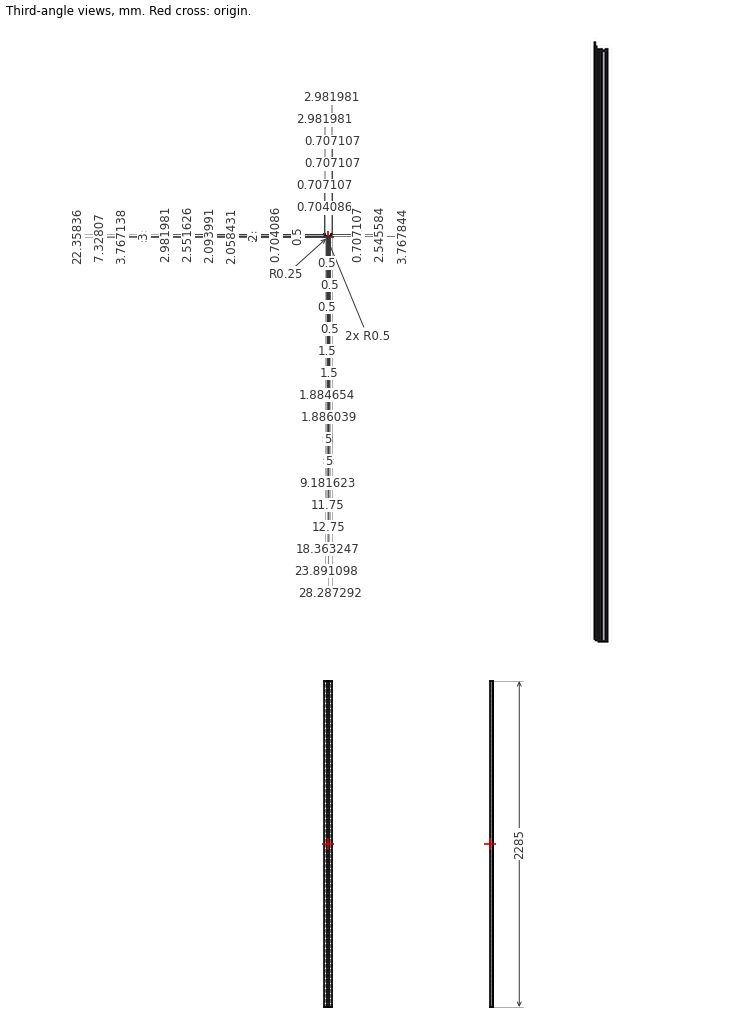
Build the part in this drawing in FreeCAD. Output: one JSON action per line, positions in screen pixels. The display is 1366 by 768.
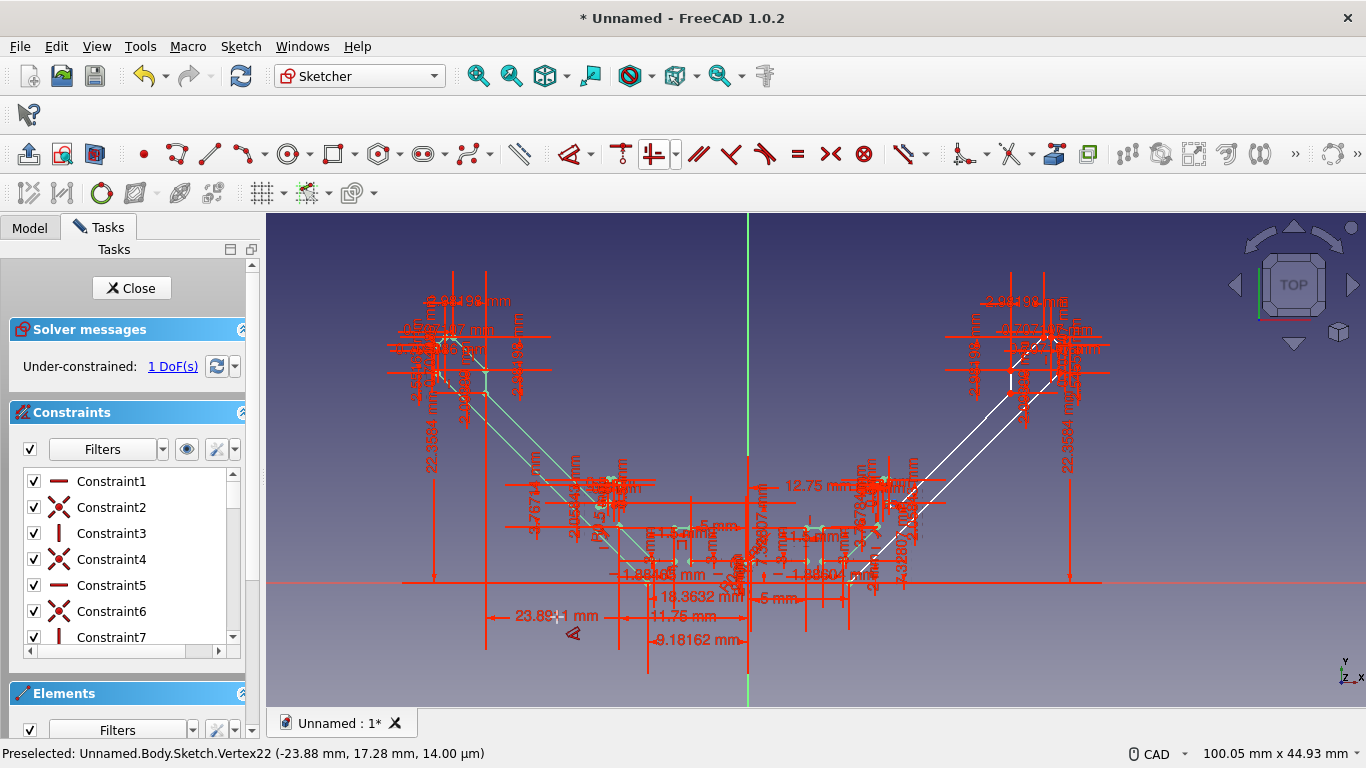
{"action": "left_click", "coordinate": [1059, 373]}
{"action": "left_click", "coordinate": [904, 617]}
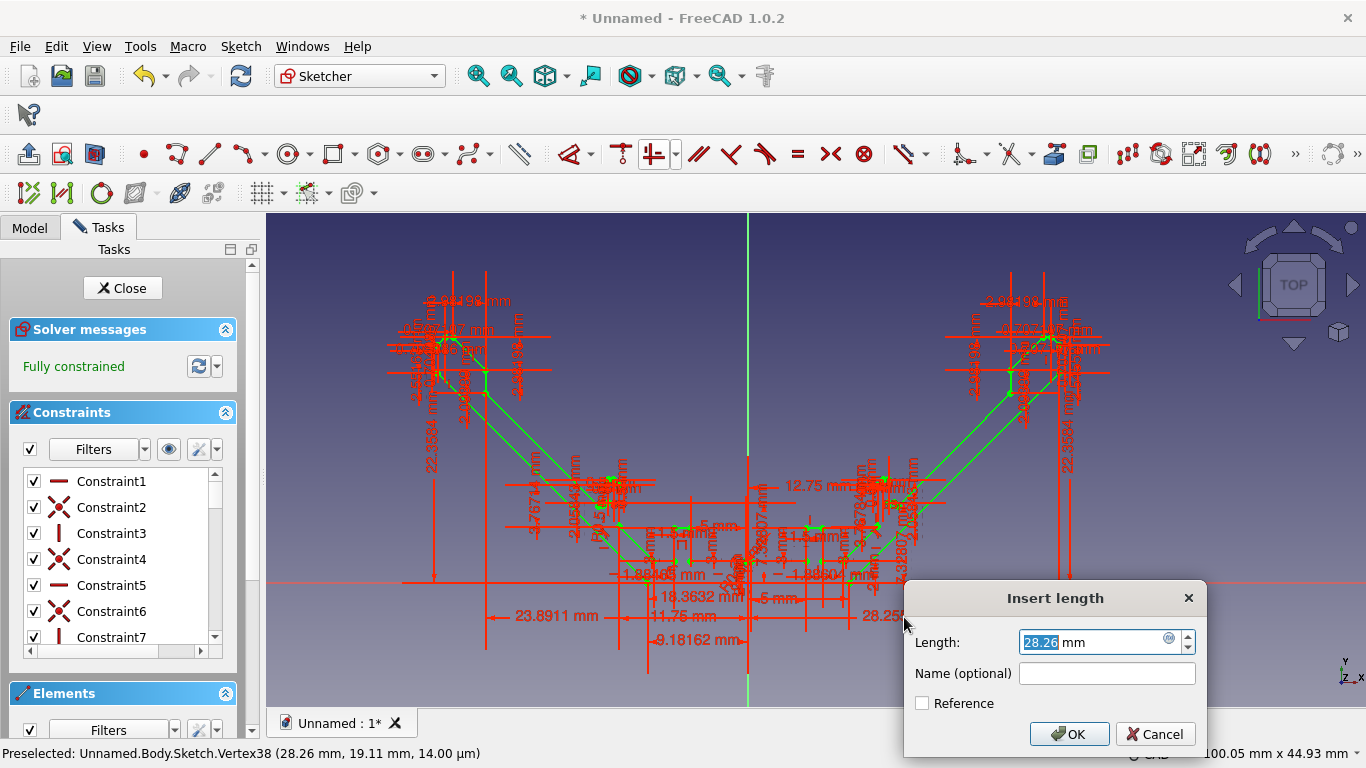
{"action": "type", "text": "28.287292"}
{"action": "key", "text": "Return"}
{"action": "key", "text": "Escape"}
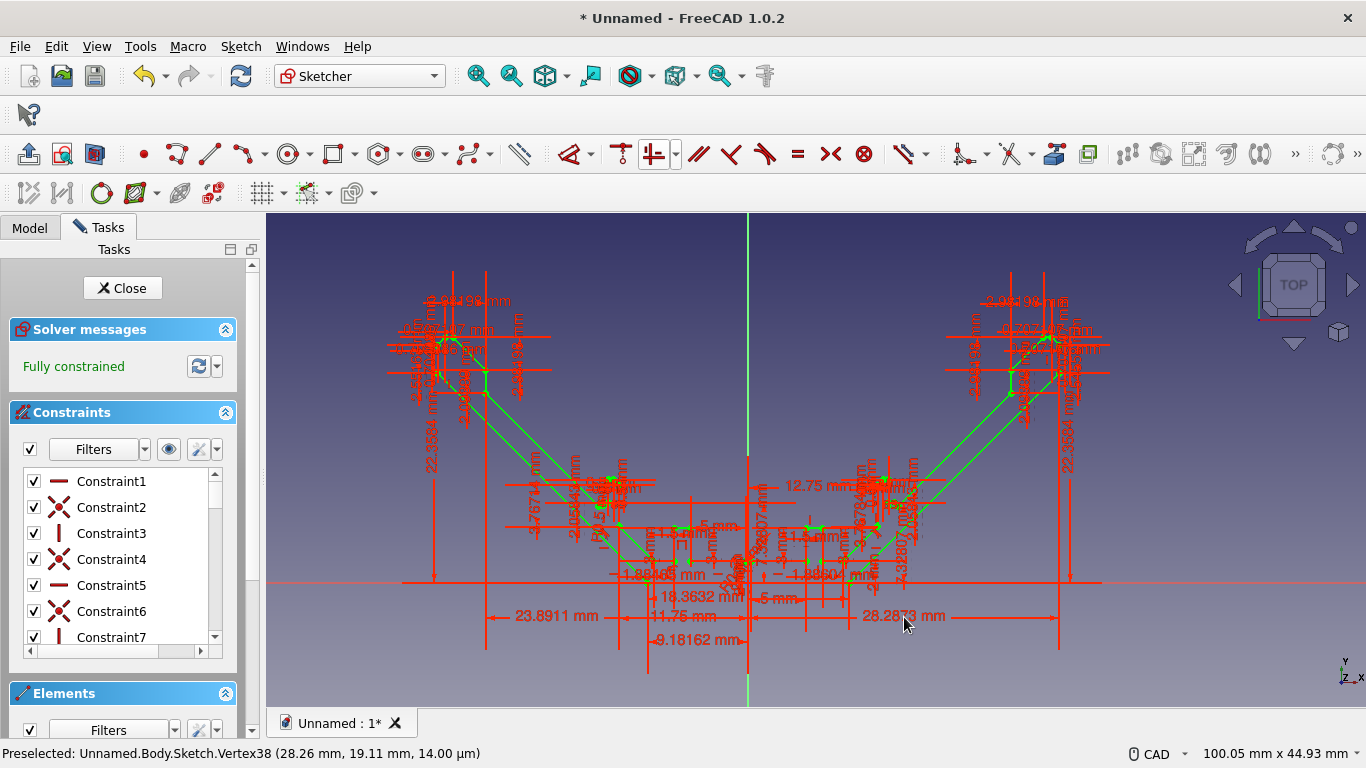
{"action": "left_click", "coordinate": [123, 288]}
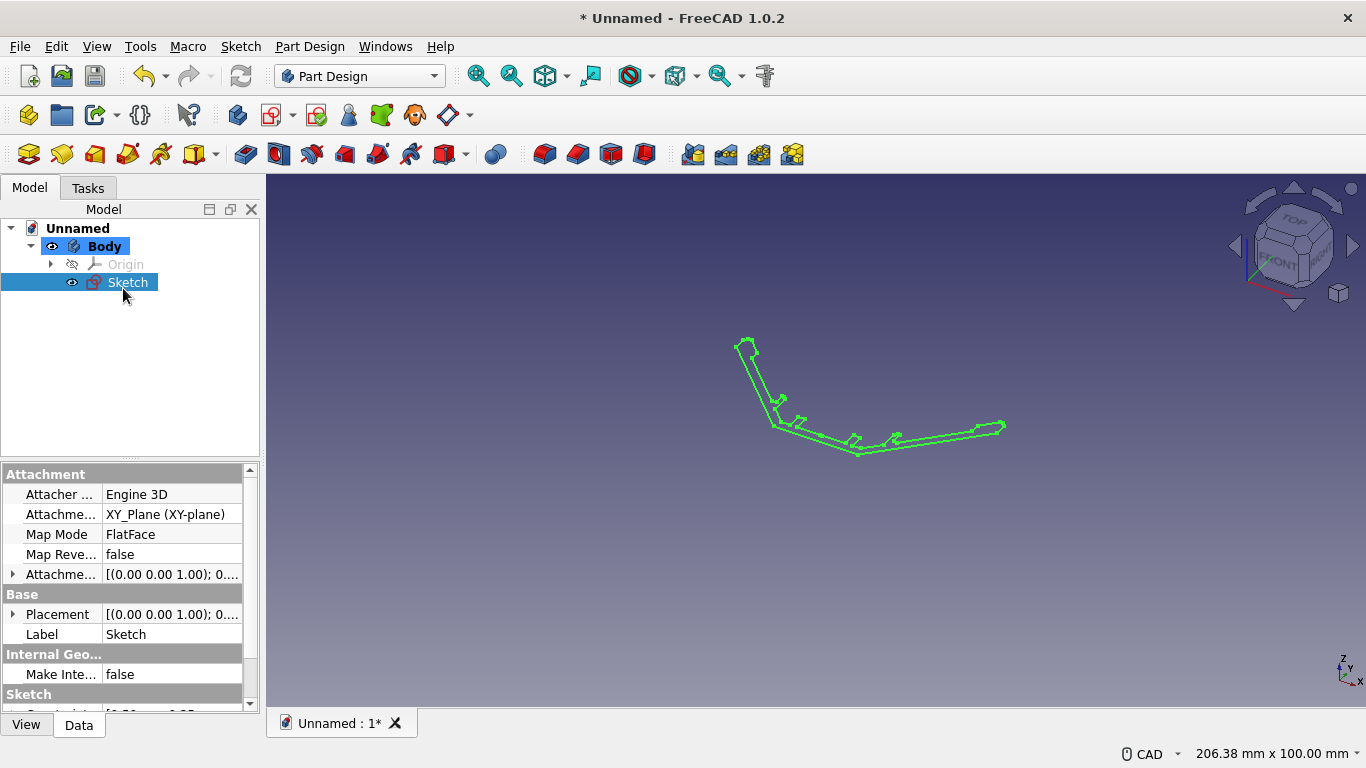
{"action": "left_click", "coordinate": [29, 154]}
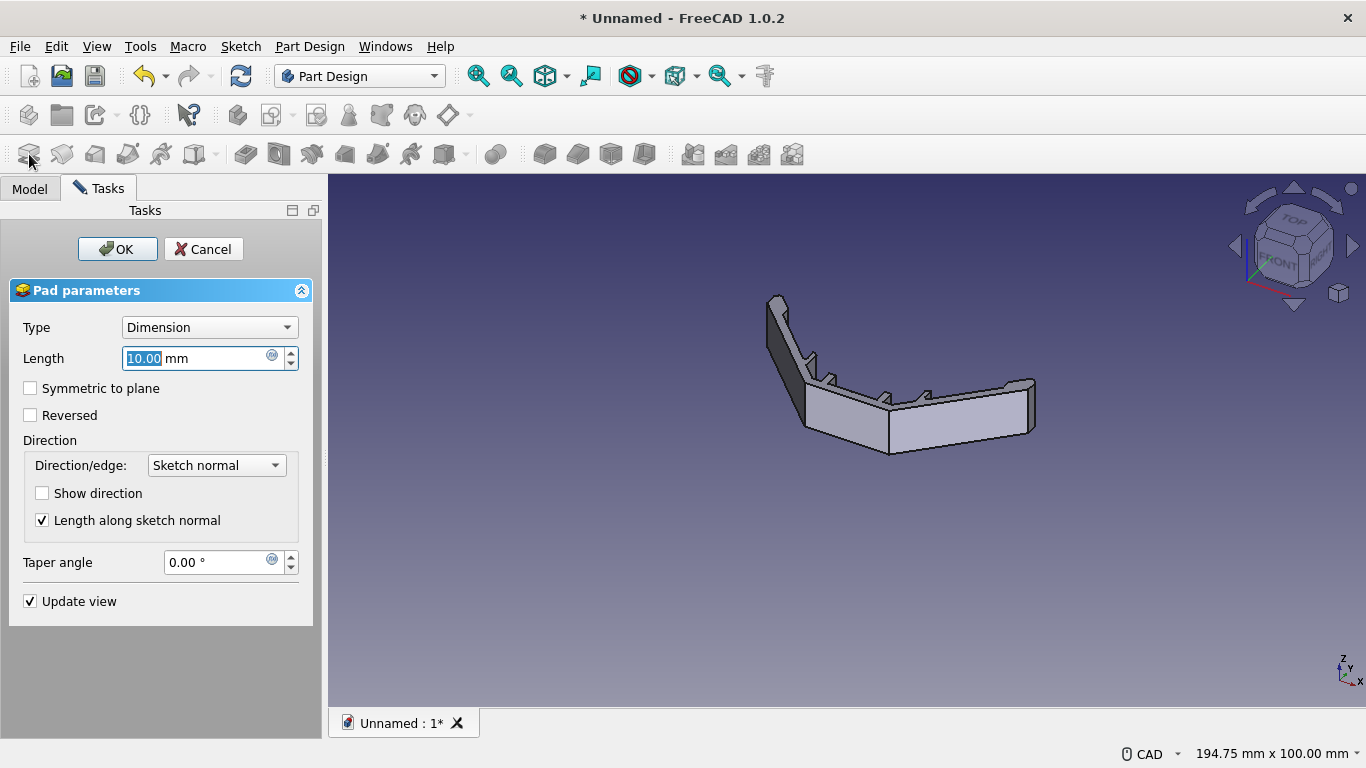
{"action": "type", "text": "2285"}
{"action": "key", "text": "Tab"}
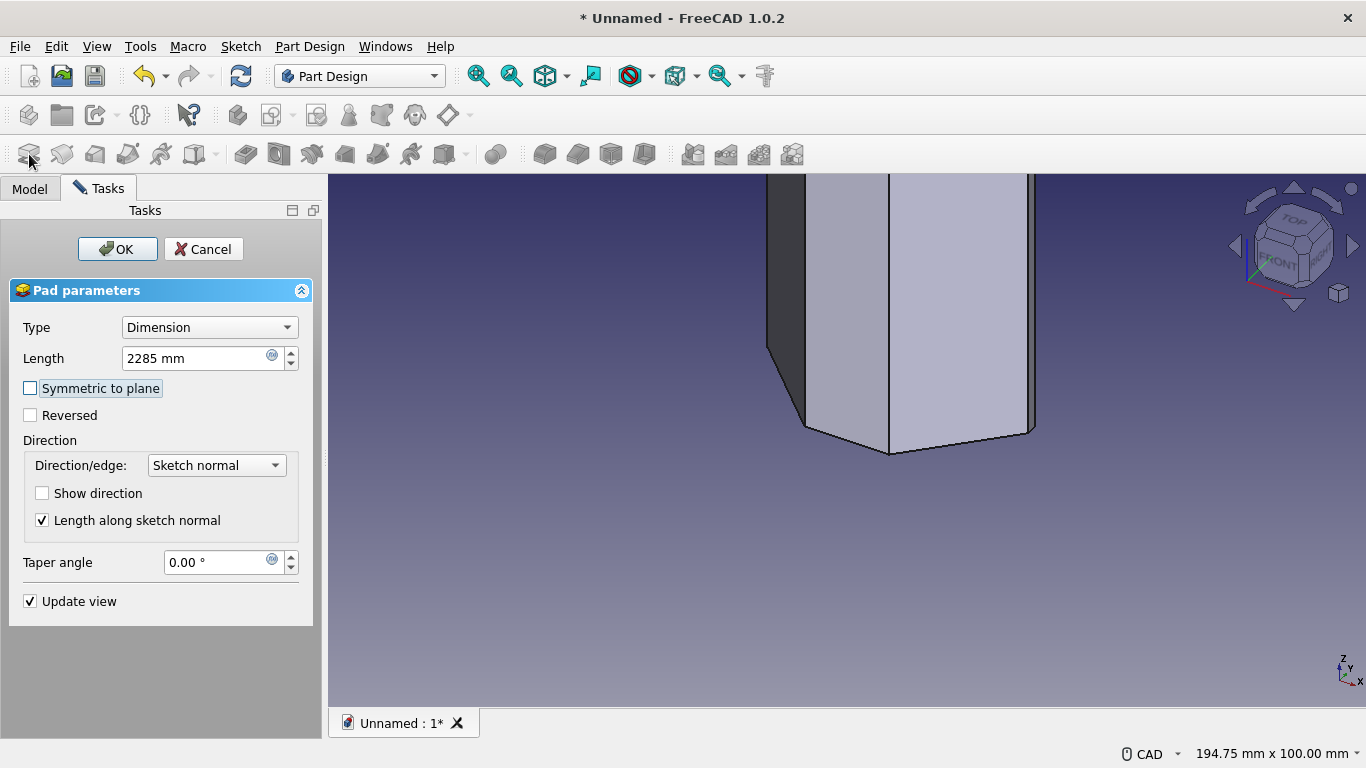
{"action": "left_click", "coordinate": [31, 388]}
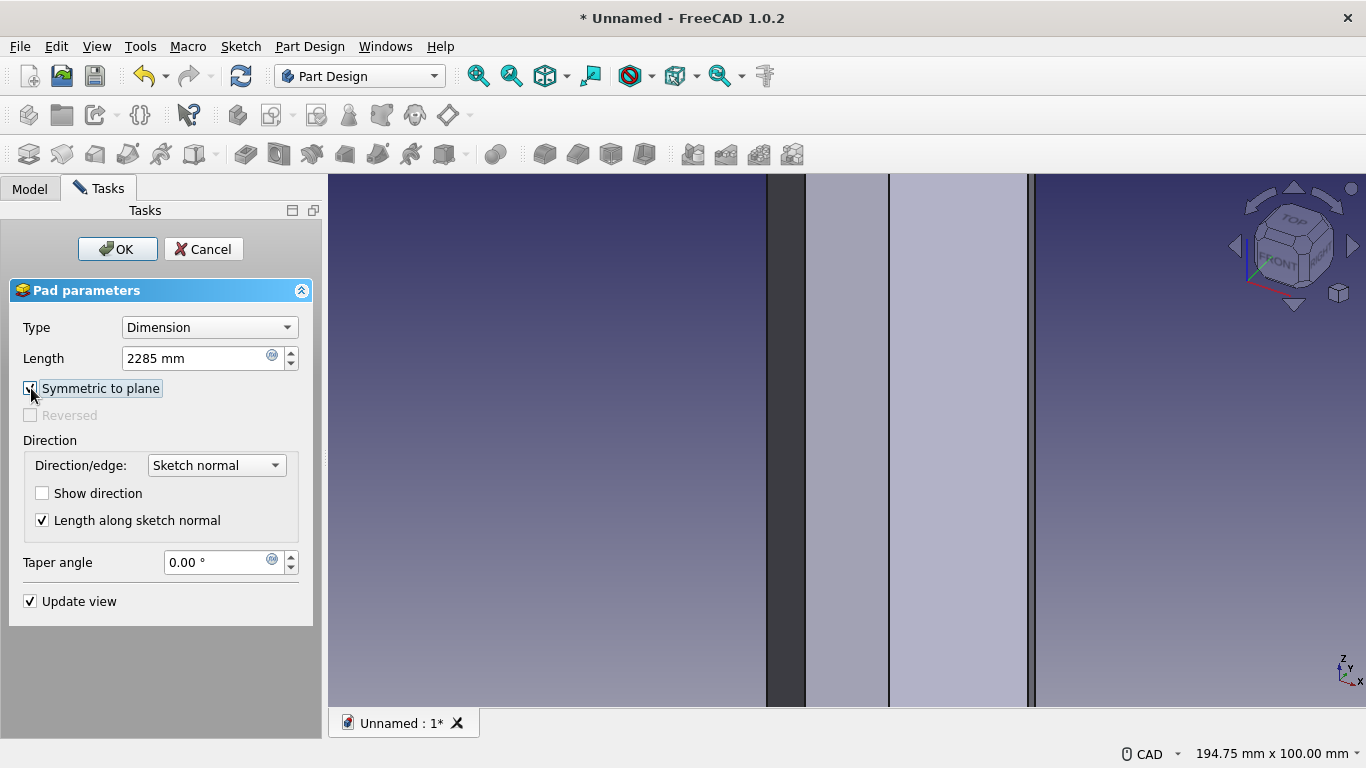
{"action": "left_click", "coordinate": [118, 249]}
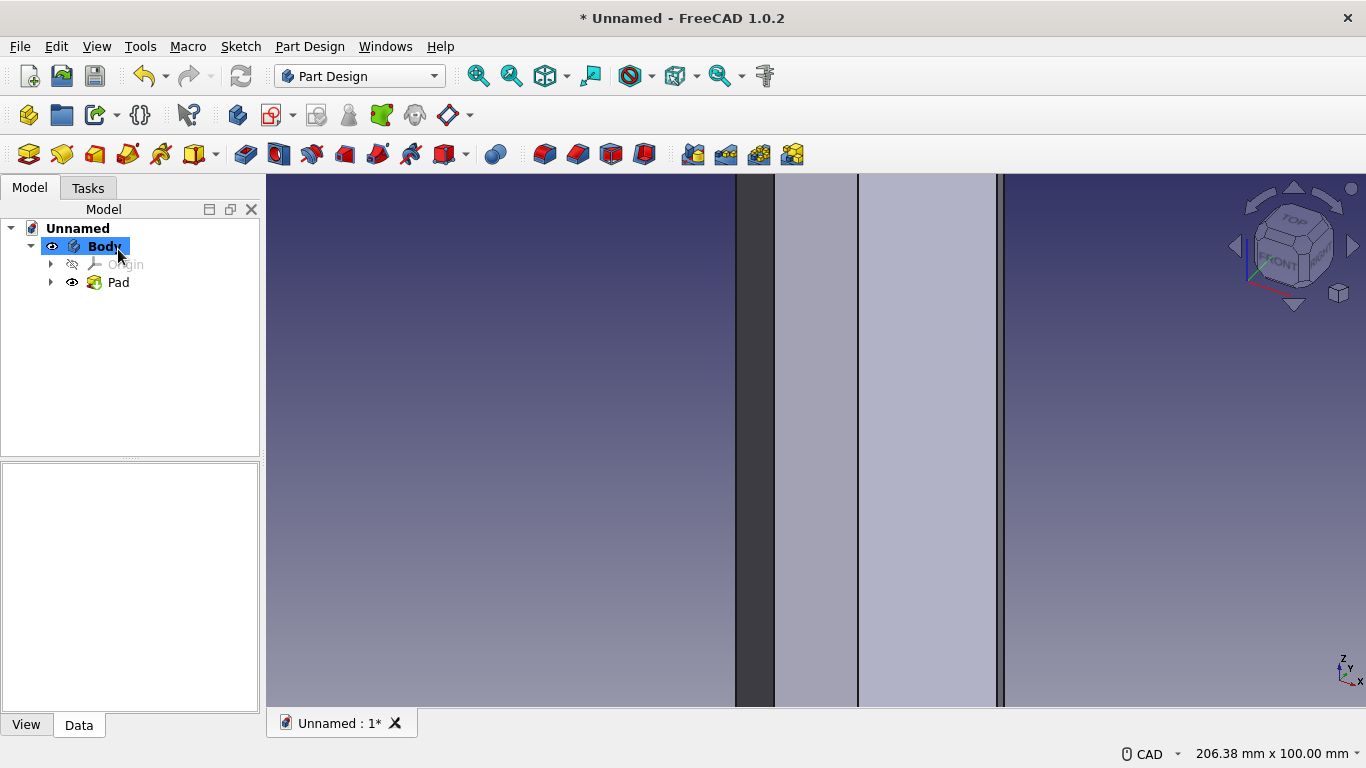
{"action": "key", "text": "0"}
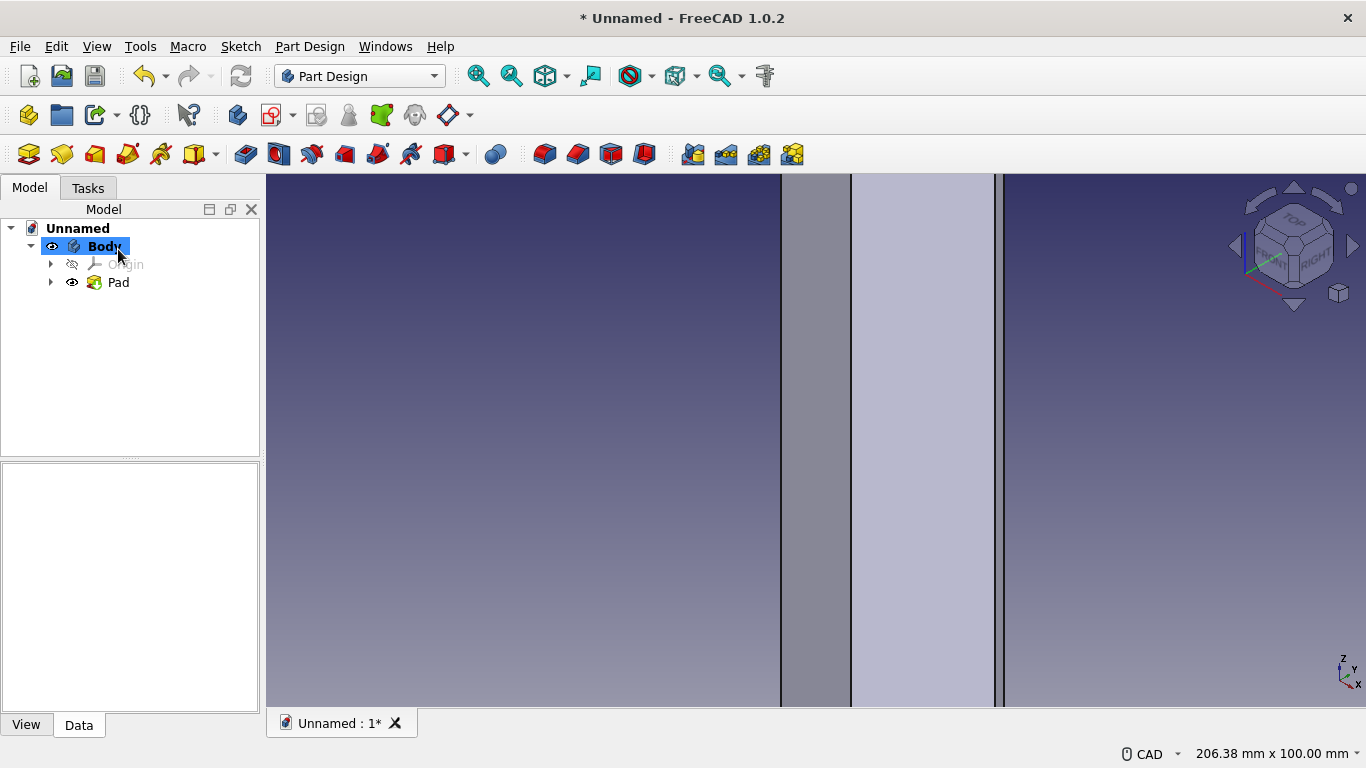
{"action": "left_click", "coordinate": [479, 76]}